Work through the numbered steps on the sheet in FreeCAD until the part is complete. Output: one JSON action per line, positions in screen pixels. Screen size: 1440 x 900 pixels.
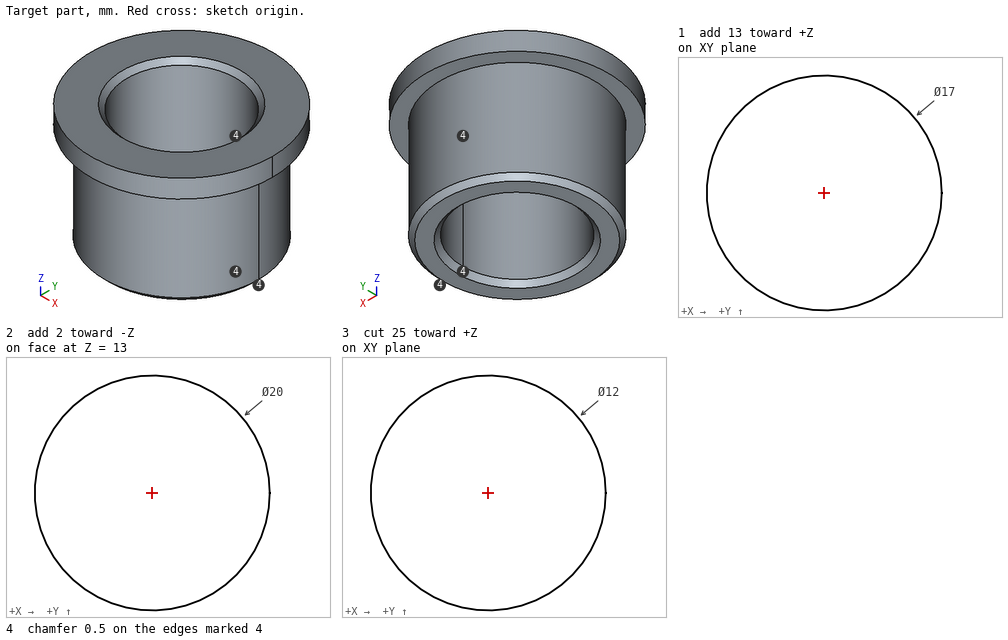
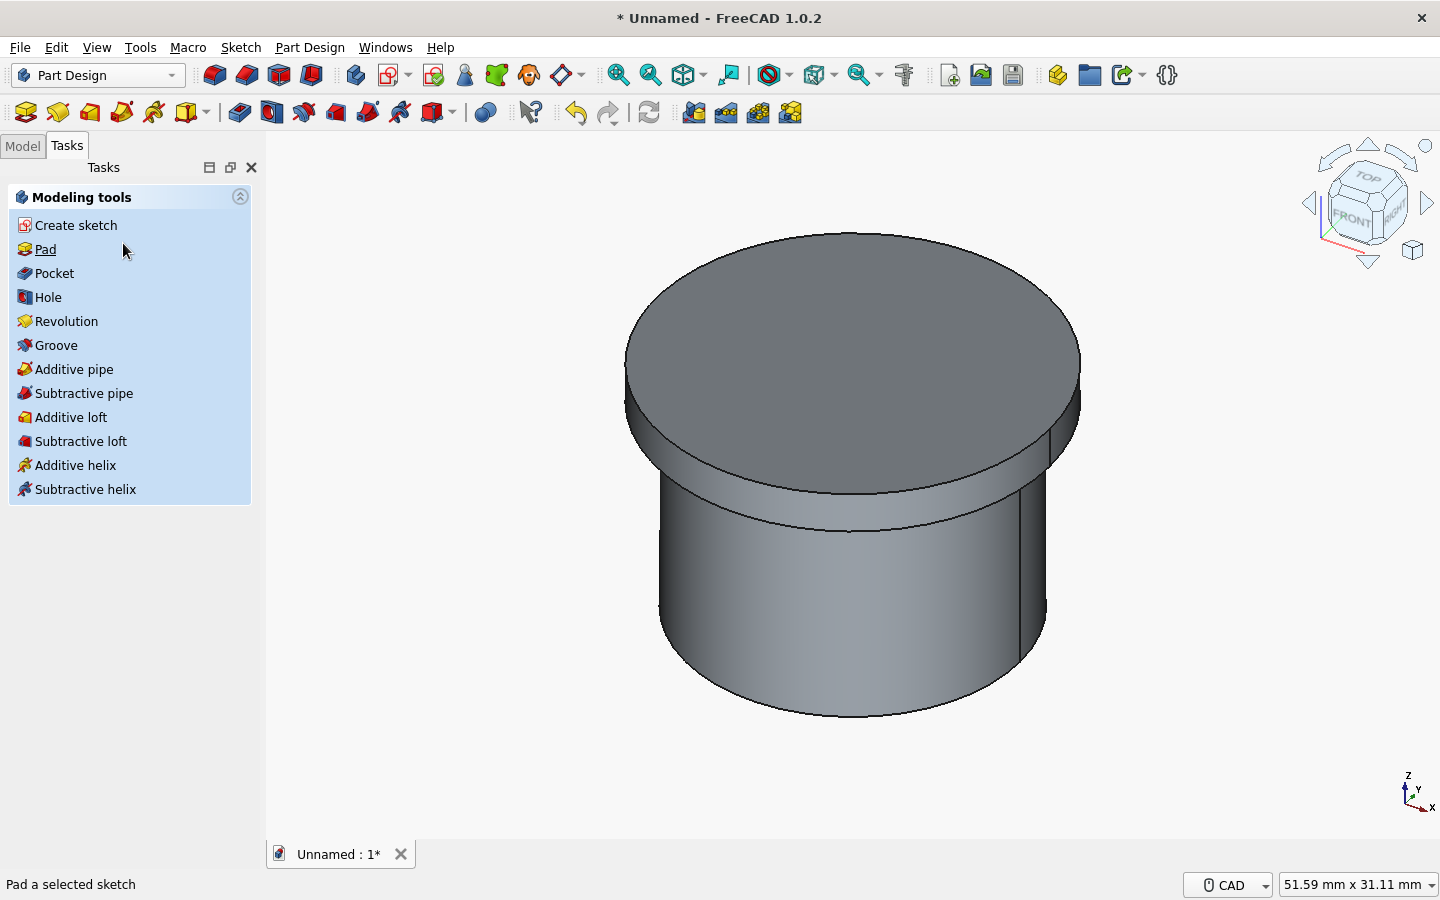
{"action": "left_click", "coordinate": [240, 112]}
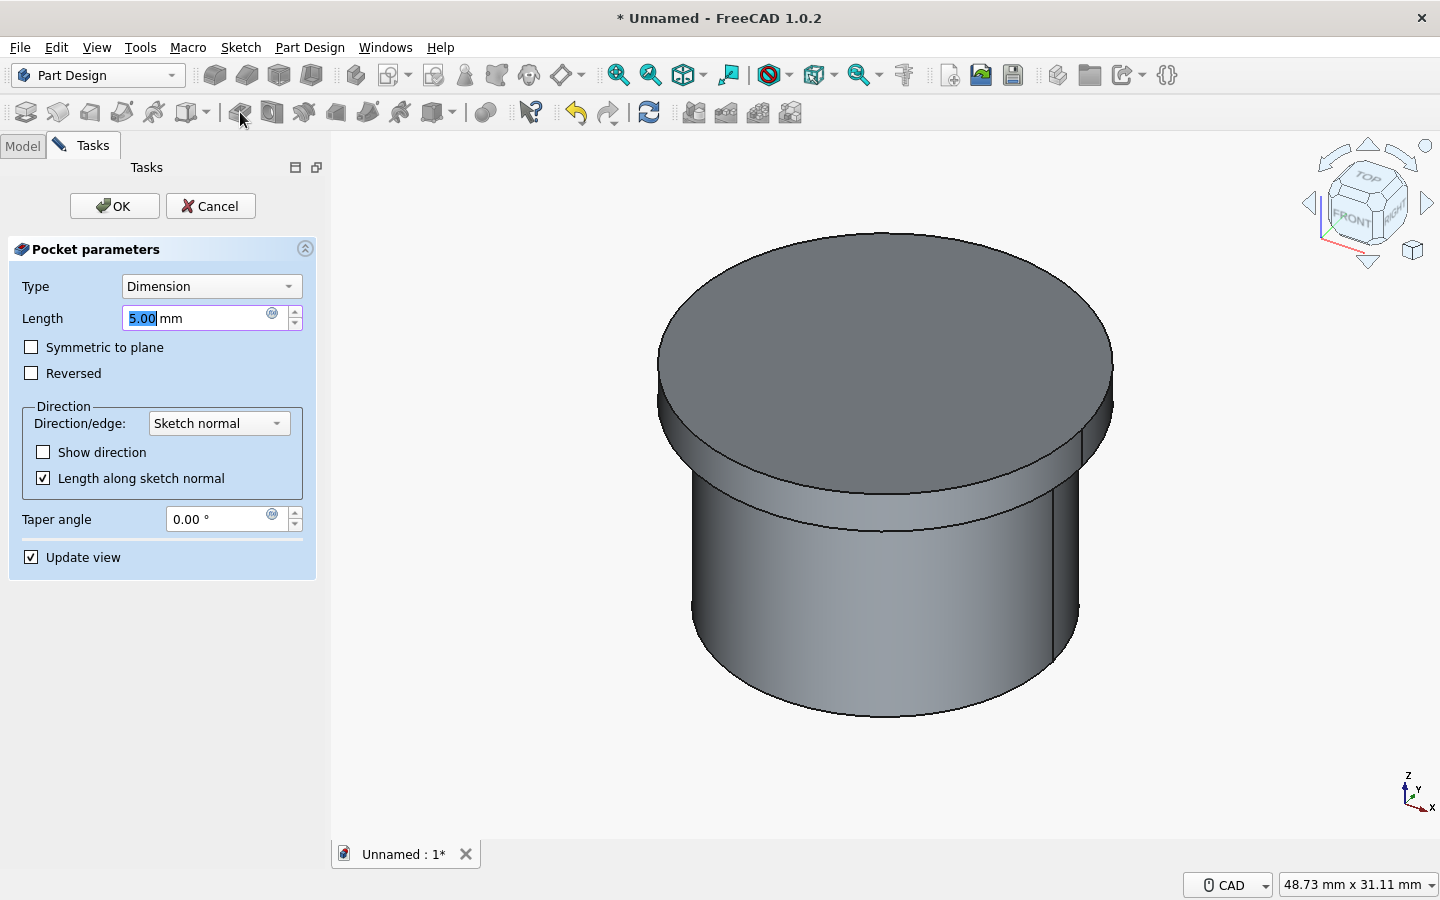
{"action": "type", "text": "25"}
{"action": "key", "text": "Tab"}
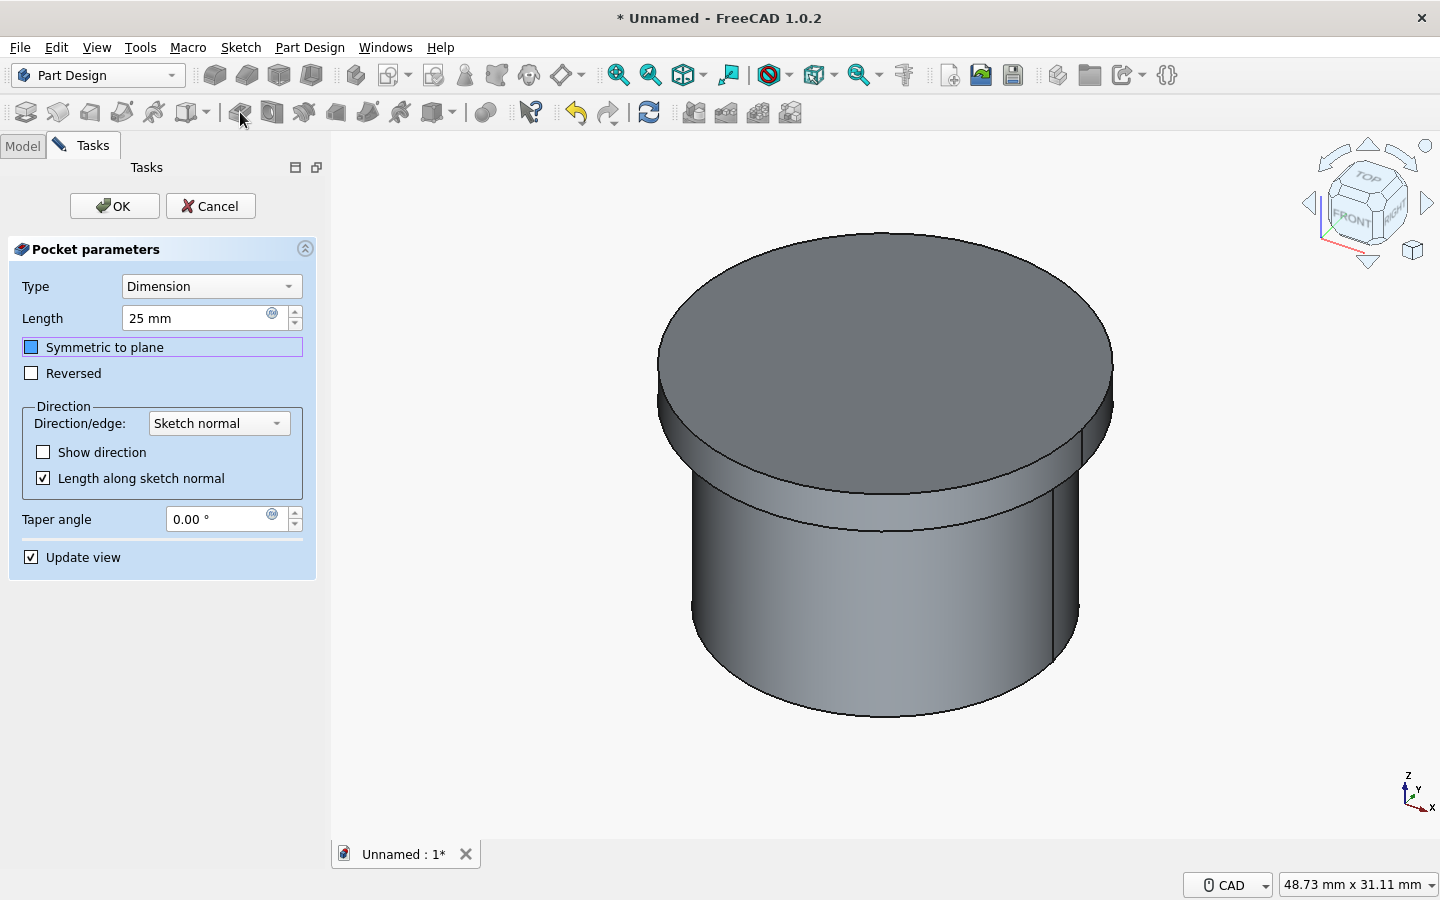
{"action": "left_click", "coordinate": [30, 373]}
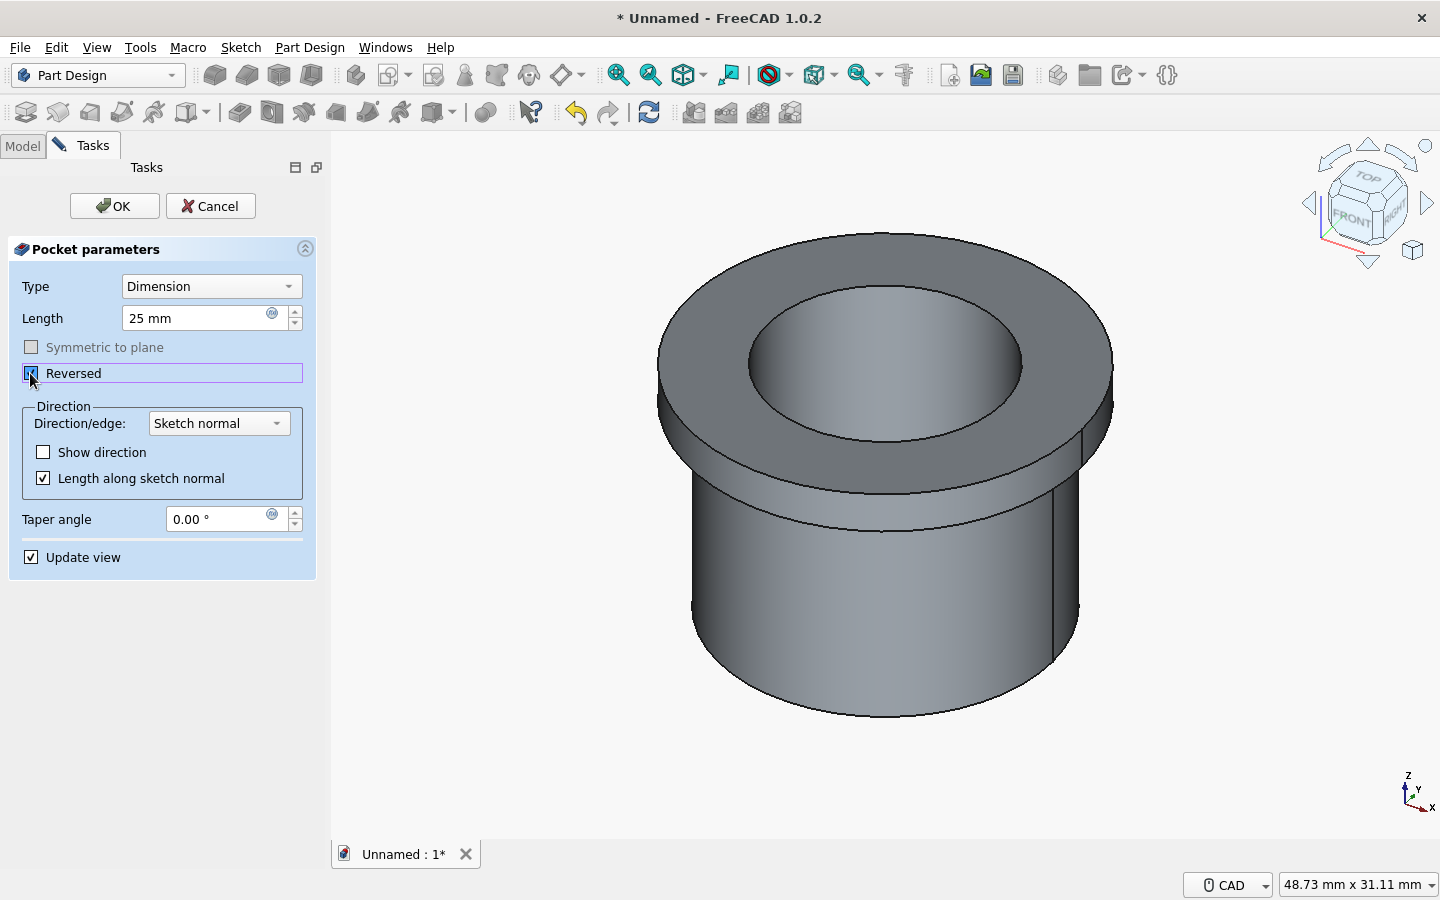
{"action": "left_click", "coordinate": [115, 206]}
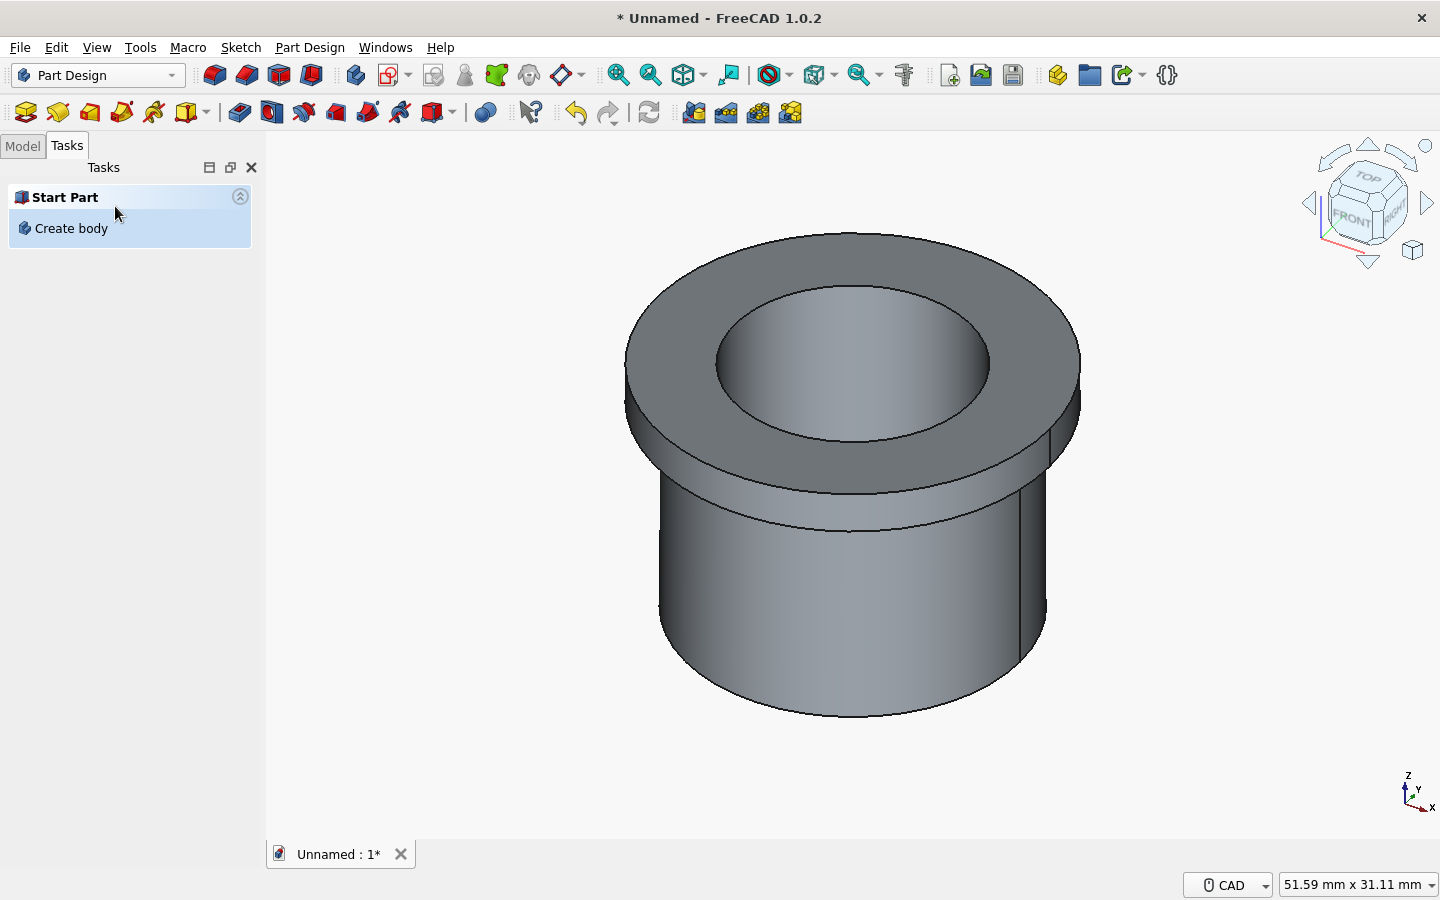
{"action": "left_click", "coordinate": [735, 324]}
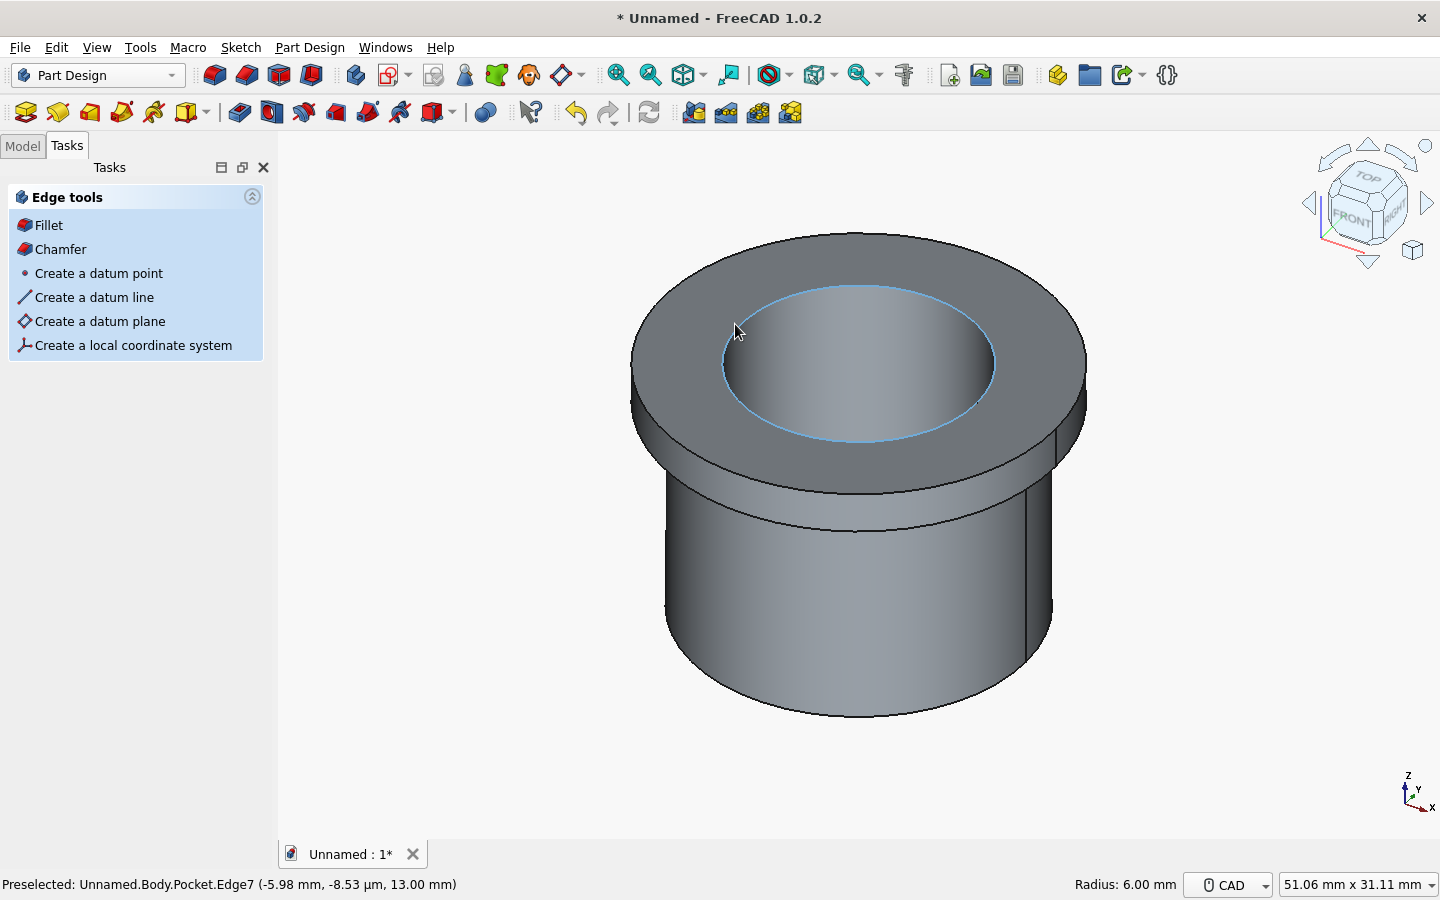
{"action": "key", "text": "0"}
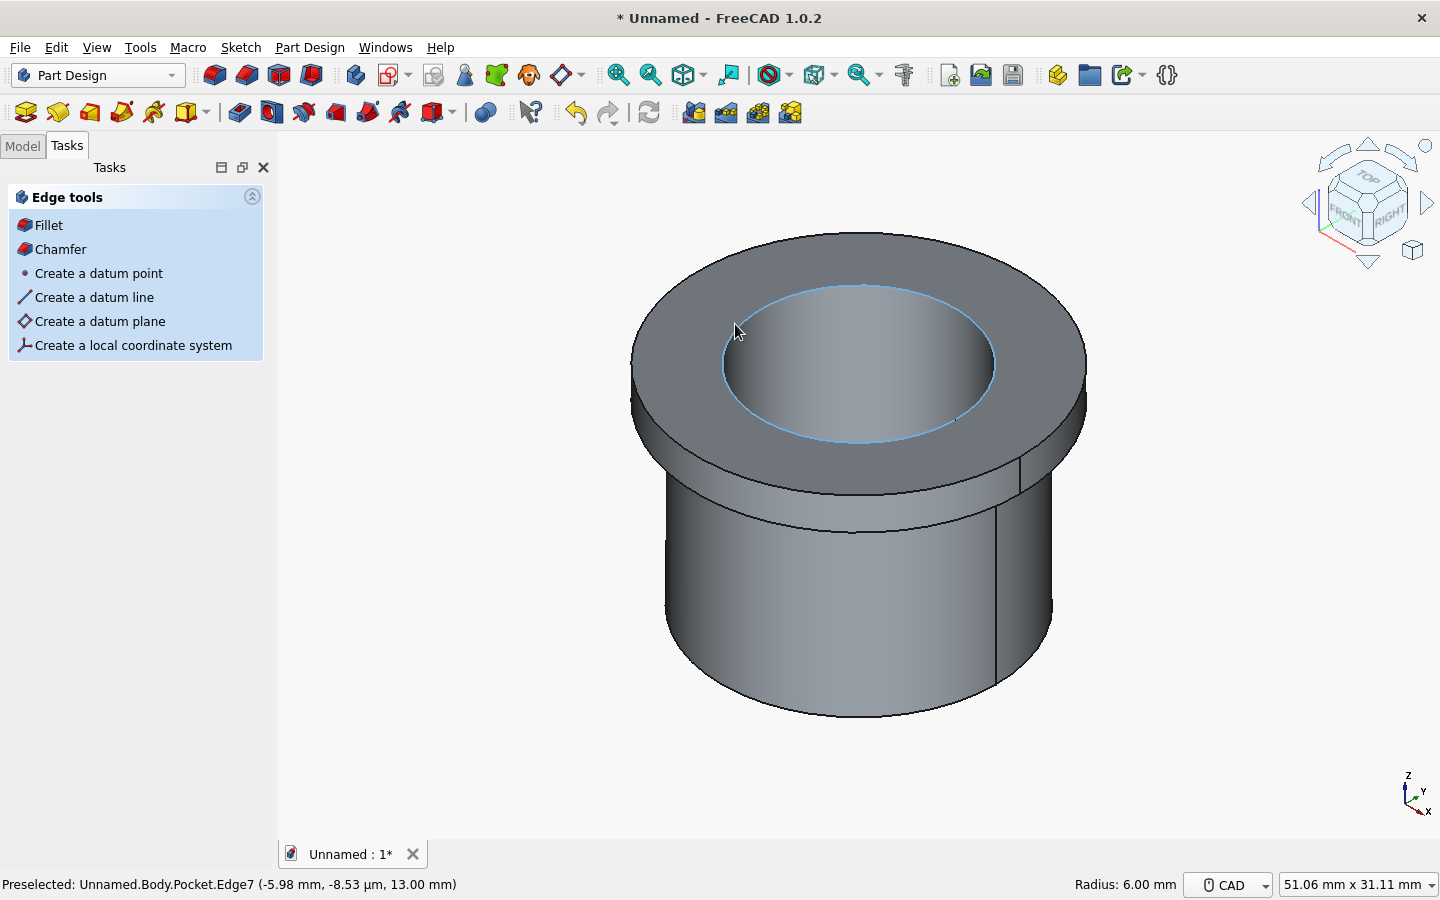
{"action": "key", "text": "2"}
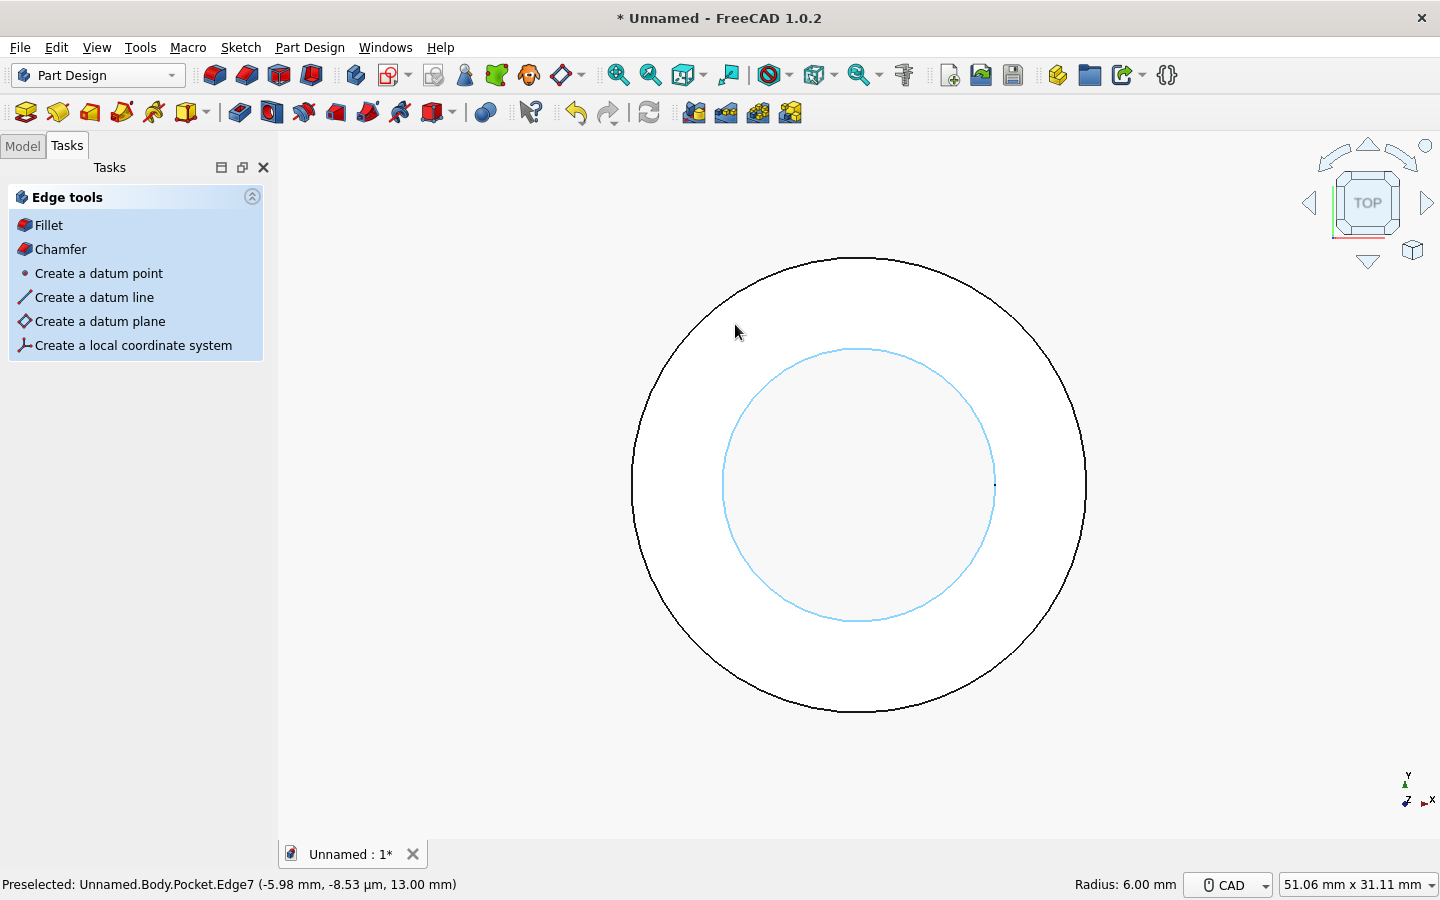
{"action": "key", "text": "1"}